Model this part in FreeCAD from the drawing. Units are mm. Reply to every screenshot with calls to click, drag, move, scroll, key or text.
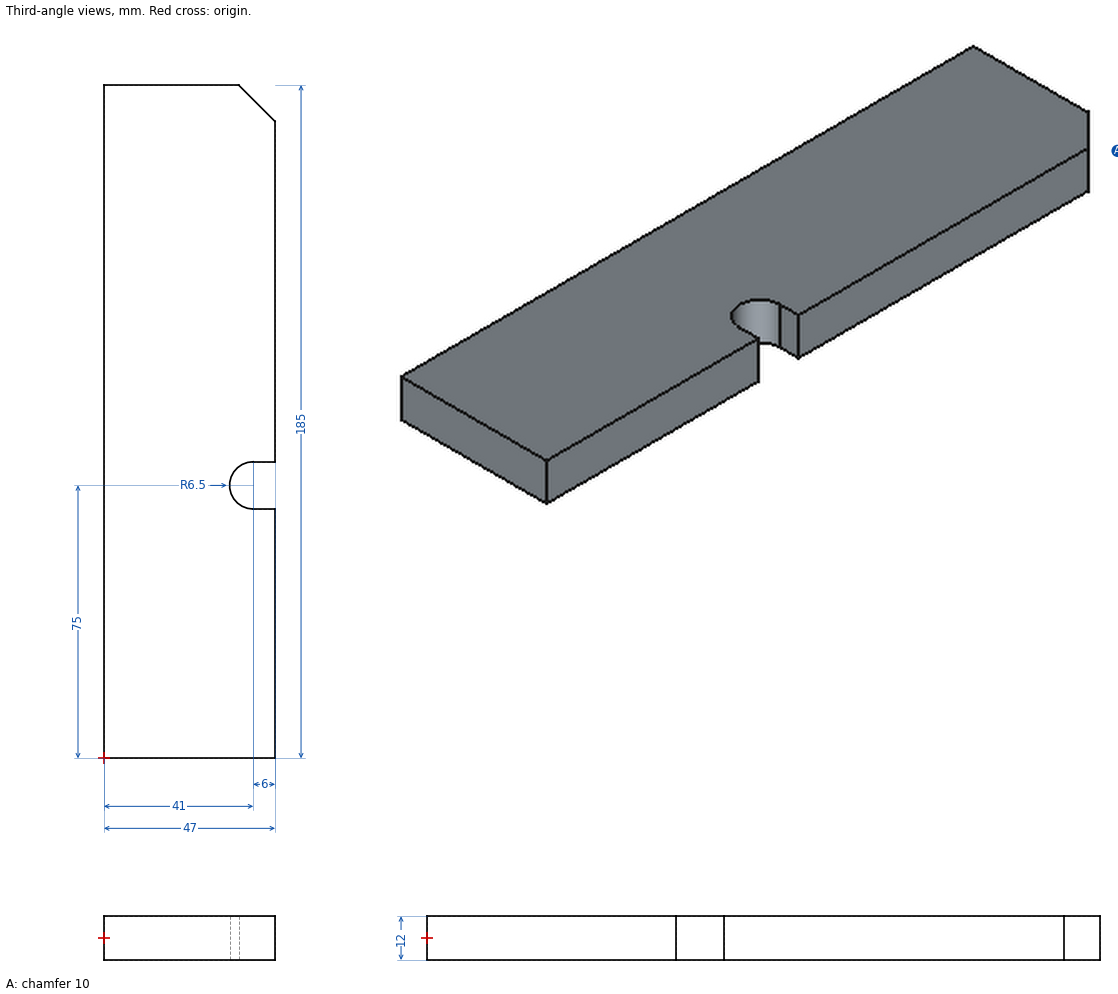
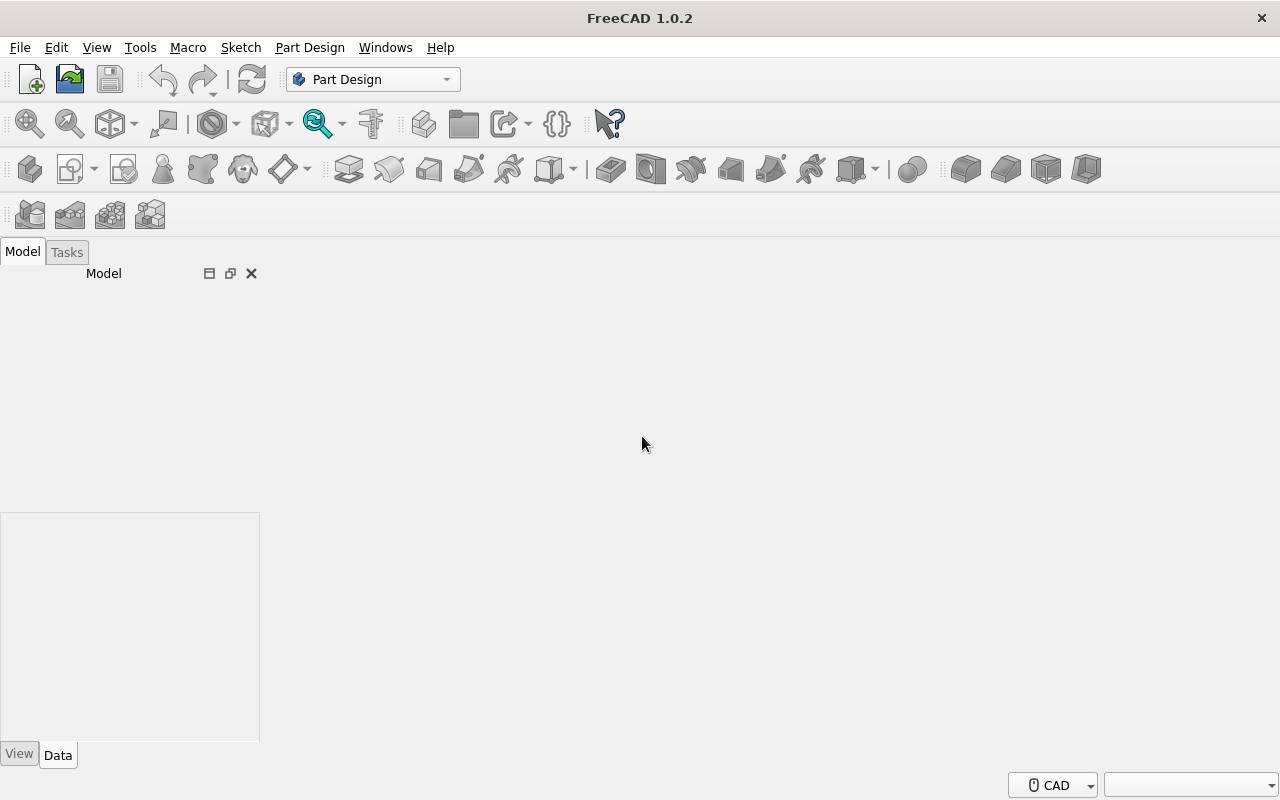
click(30, 80)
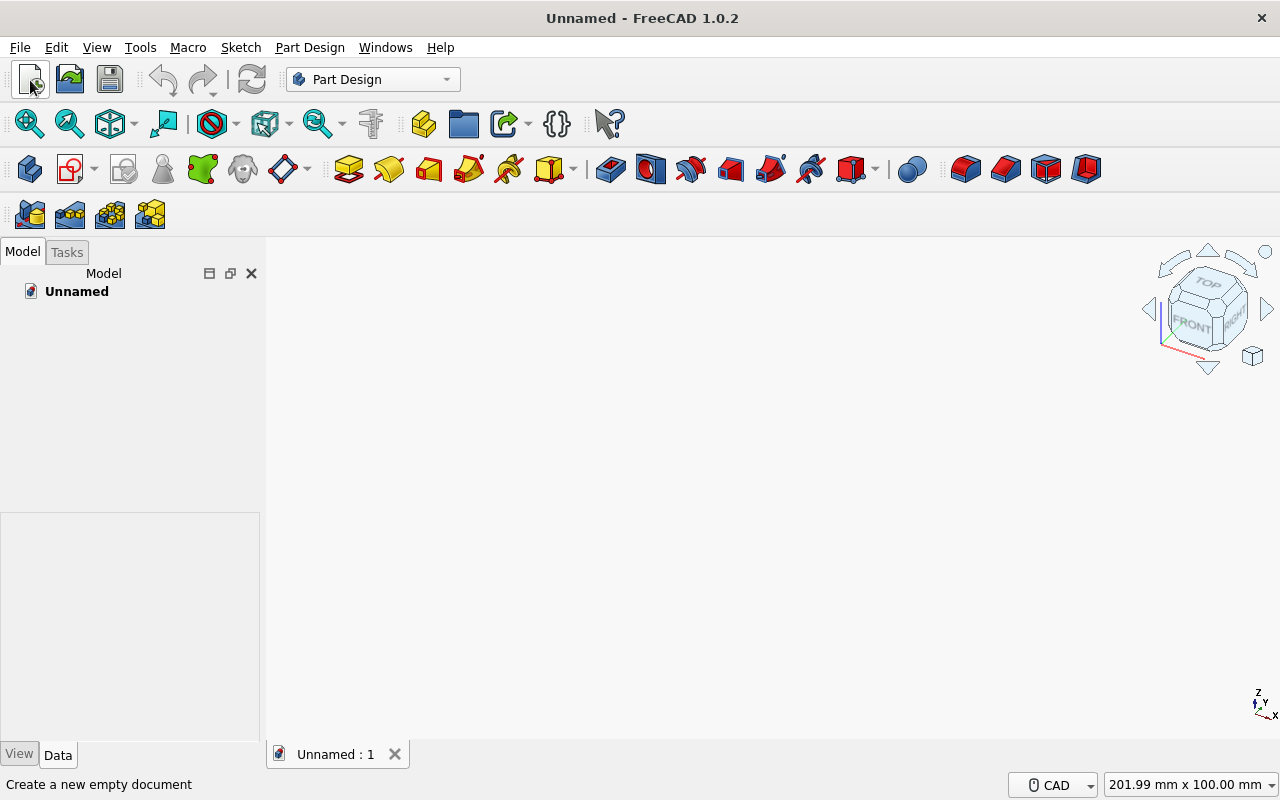
click(70, 170)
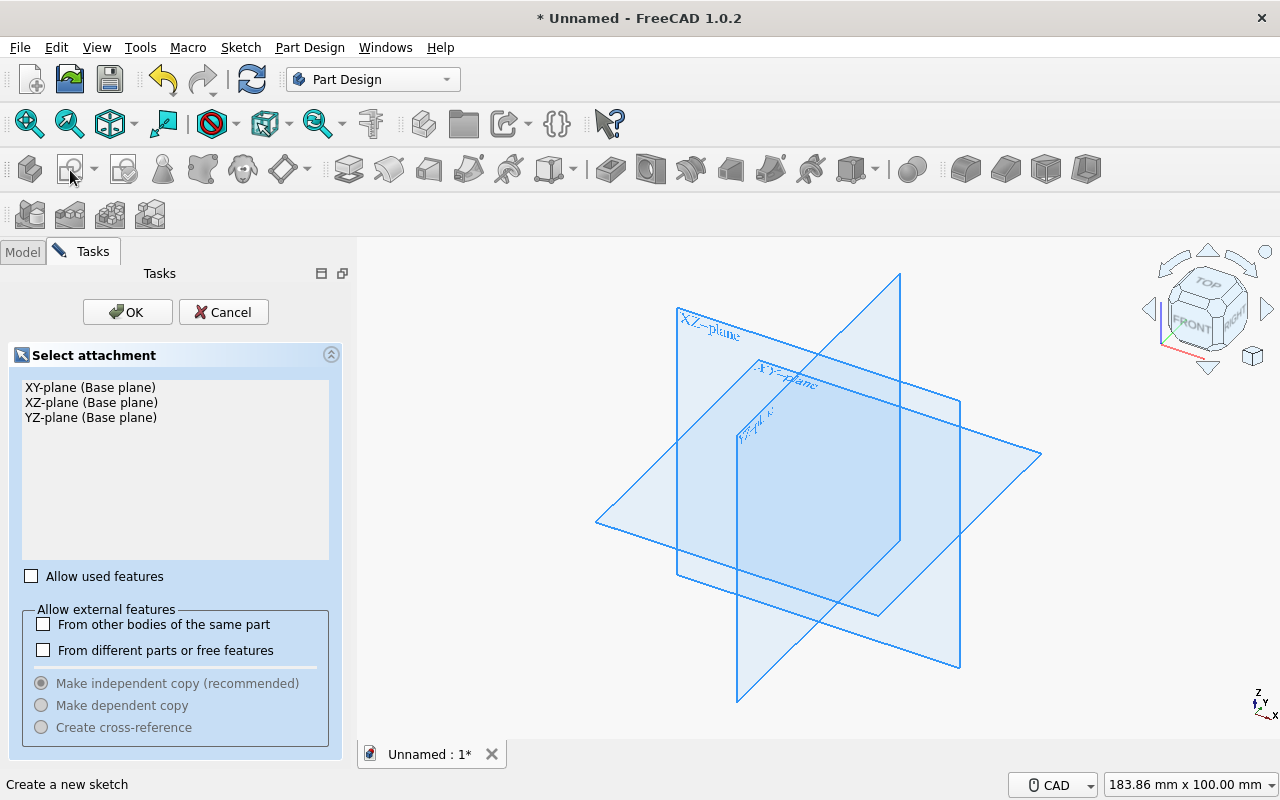
click(82, 388)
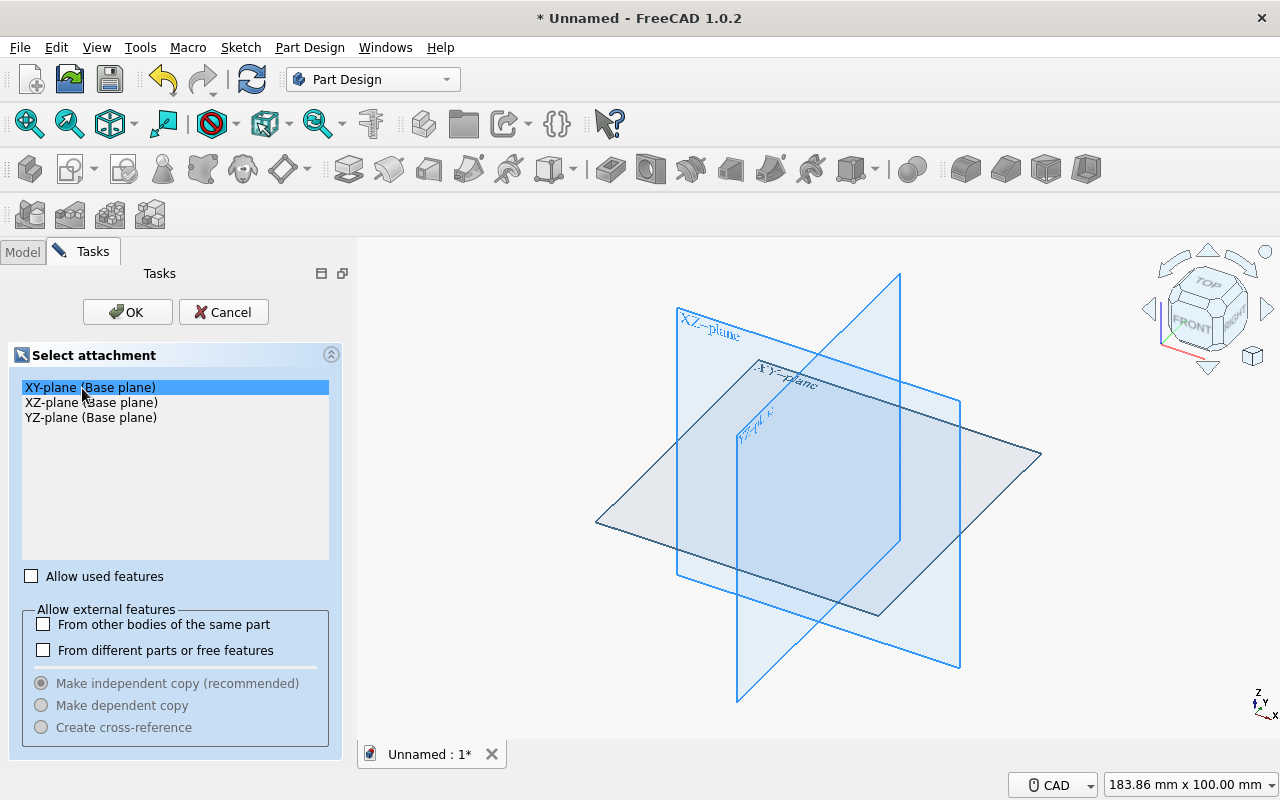
click(128, 312)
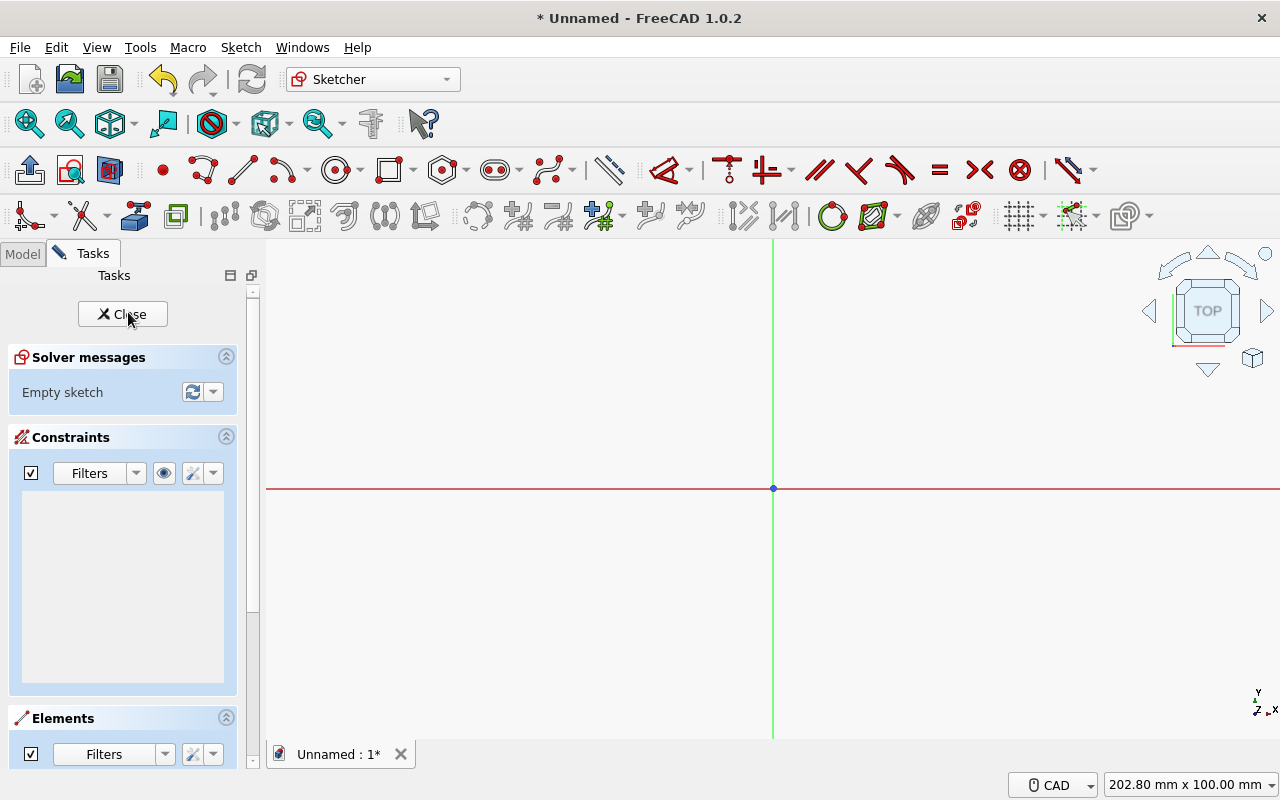
scroll(624, 688, down, 6)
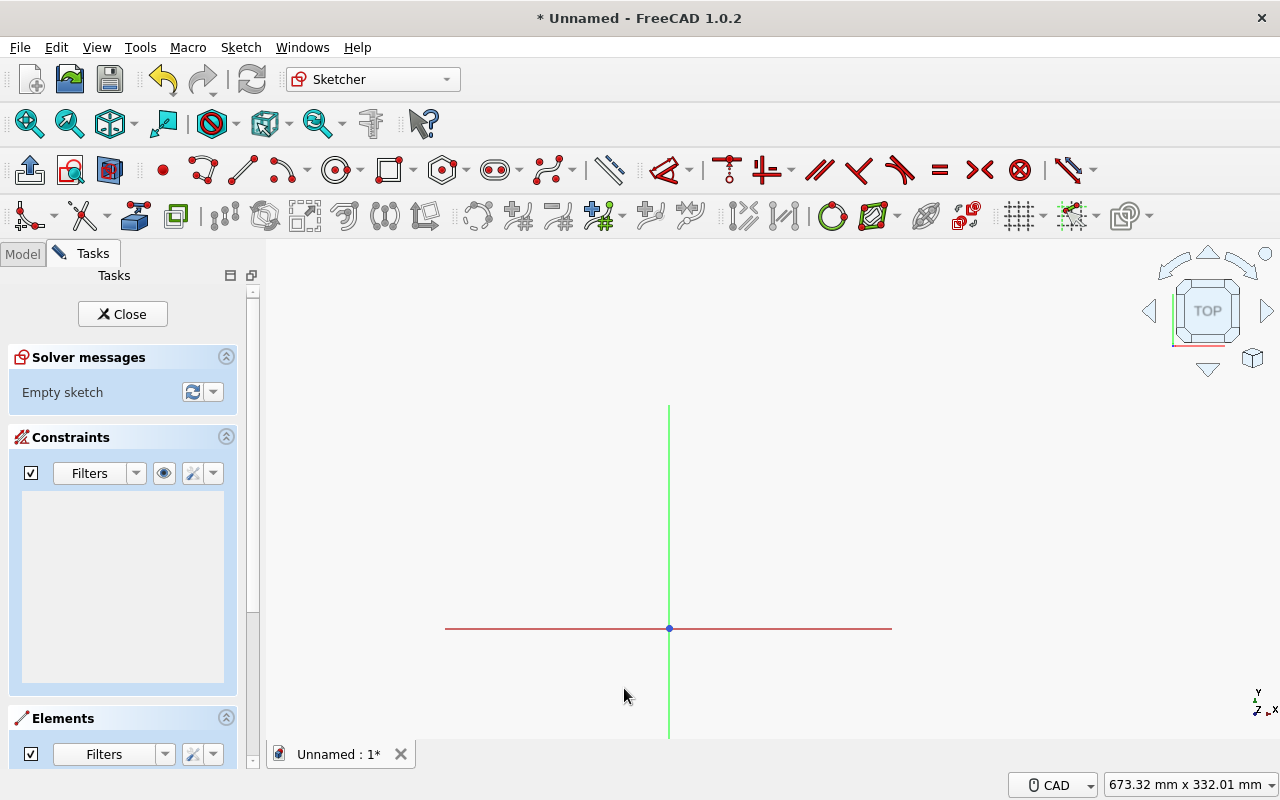
click(390, 170)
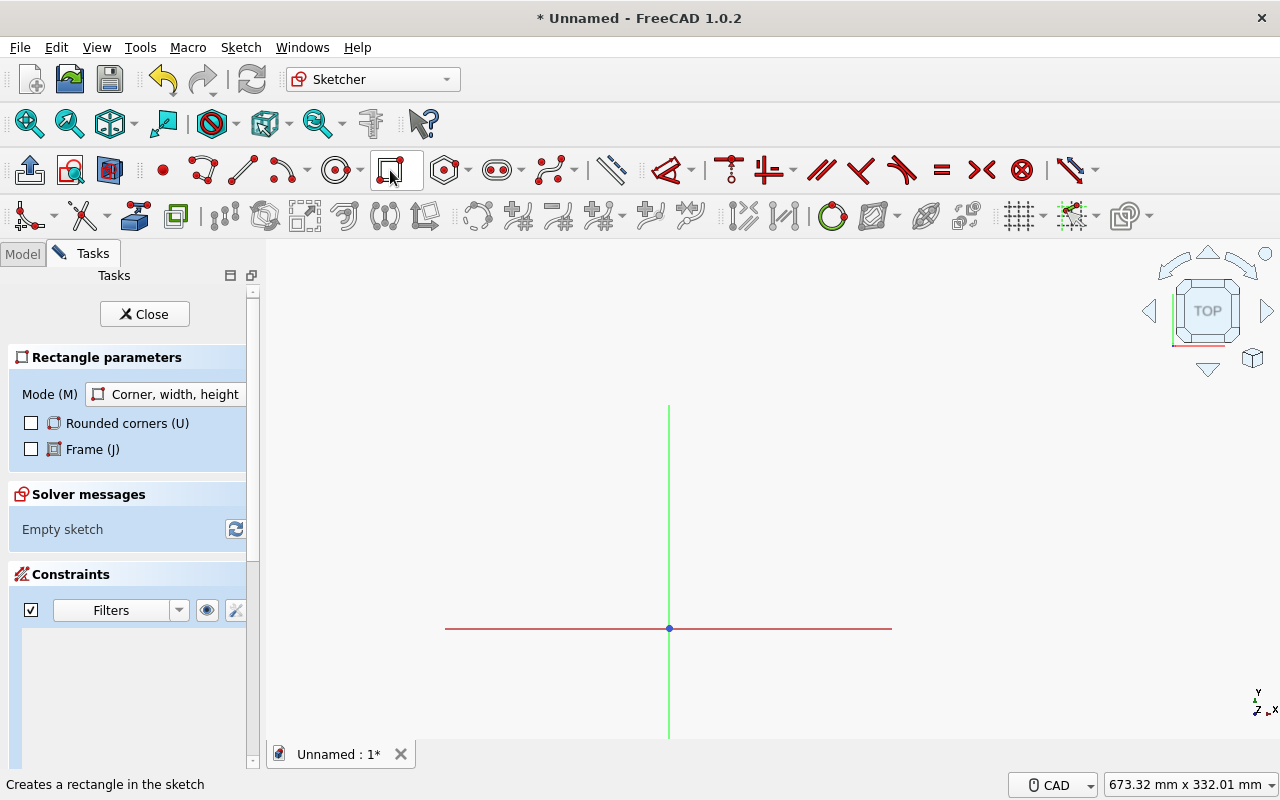
click(669, 629)
click(740, 350)
key(Escape)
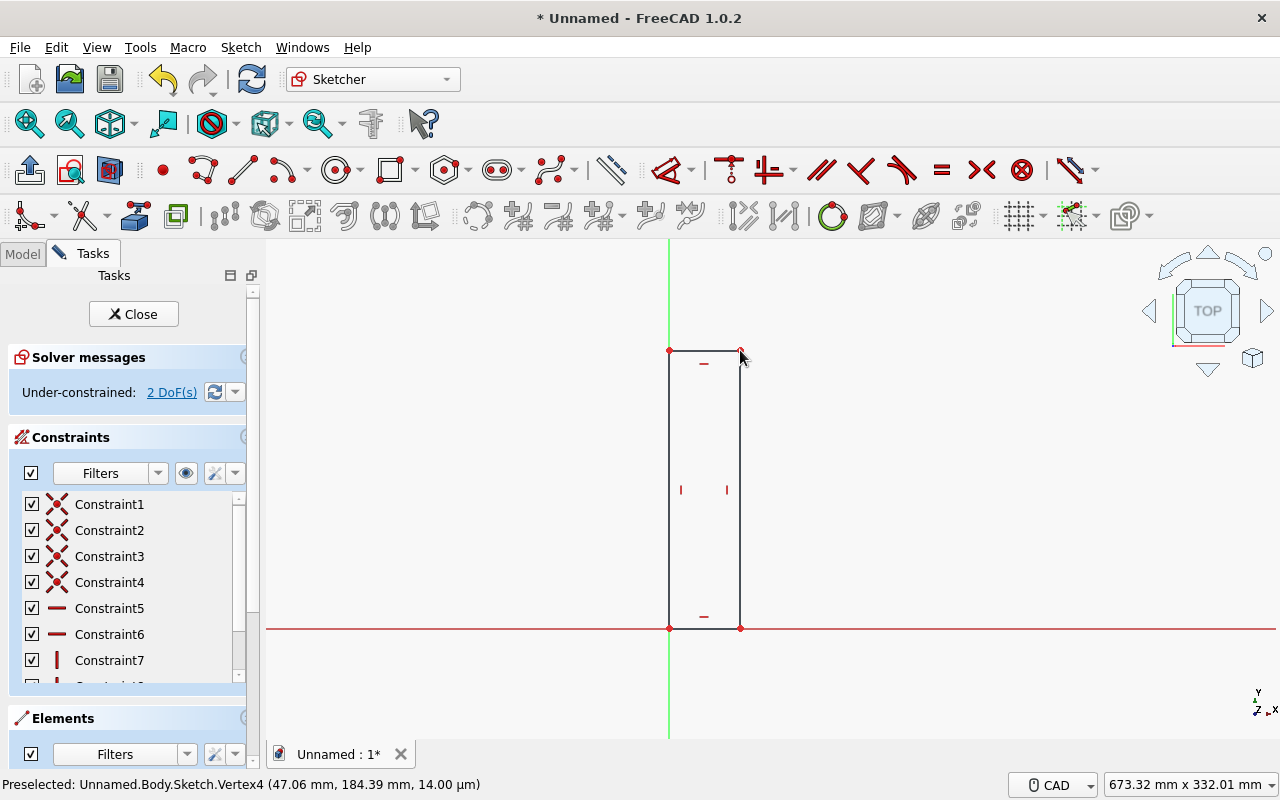
click(666, 170)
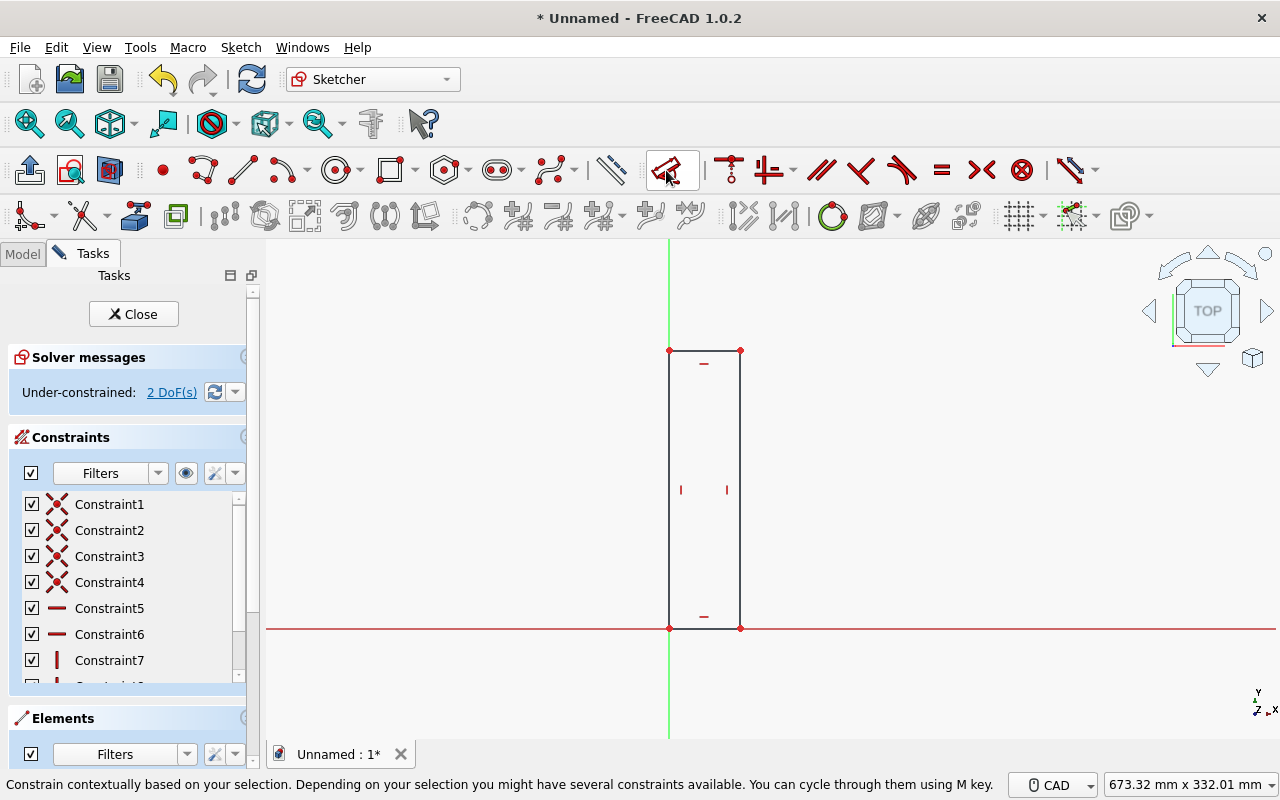
click(690, 629)
click(705, 663)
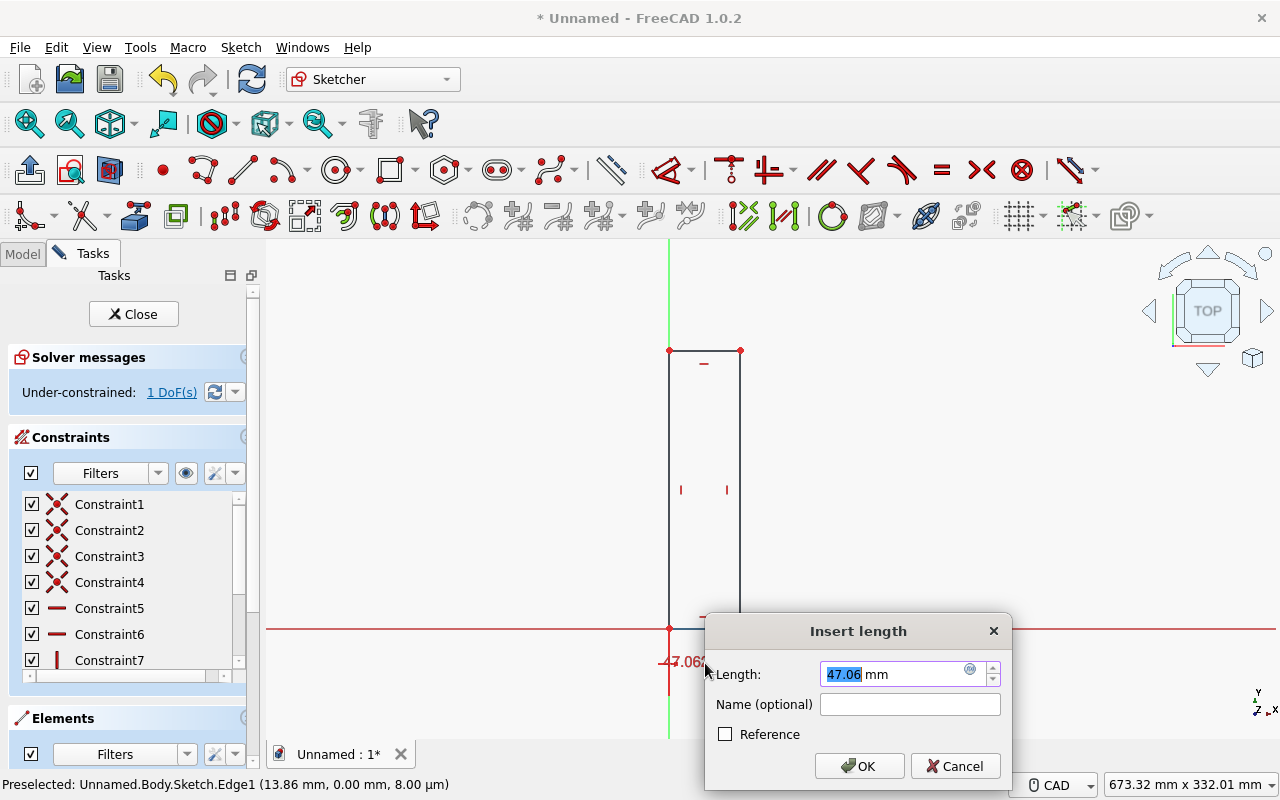
text(47)
key(Return)